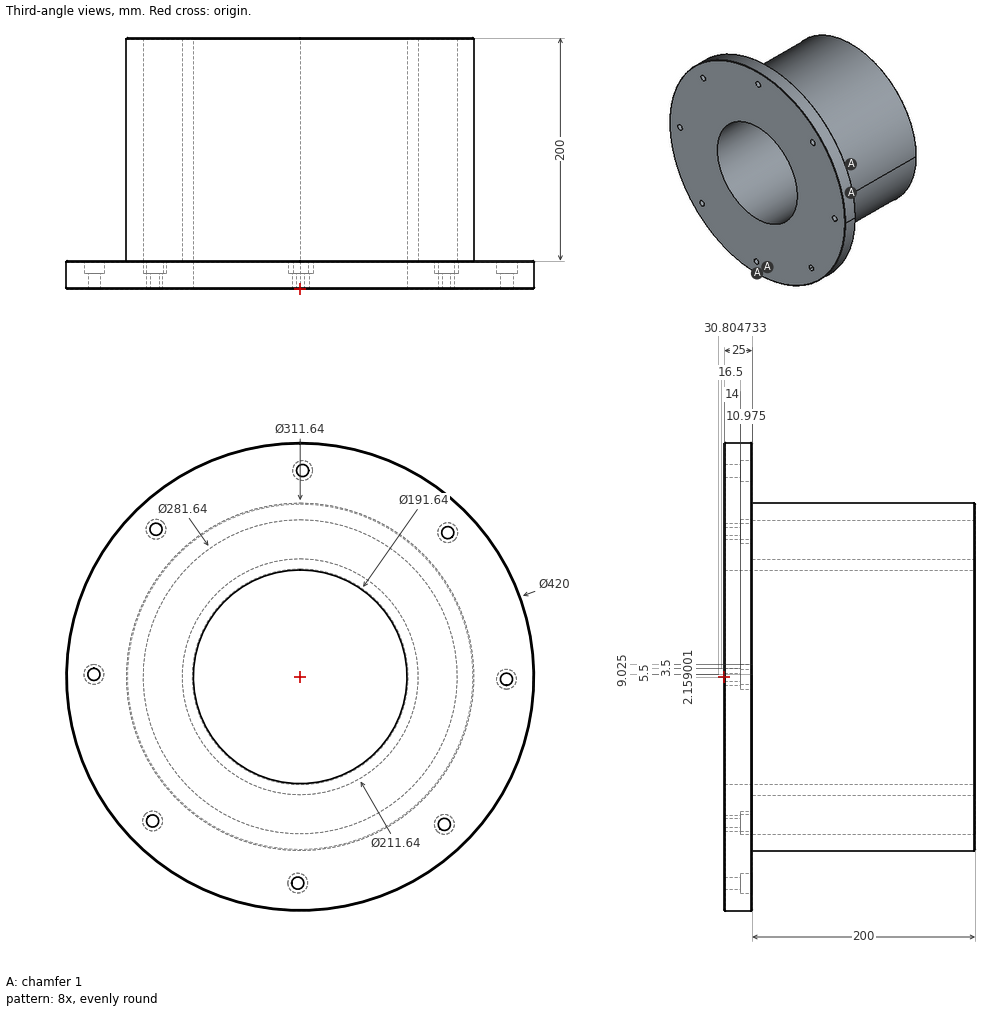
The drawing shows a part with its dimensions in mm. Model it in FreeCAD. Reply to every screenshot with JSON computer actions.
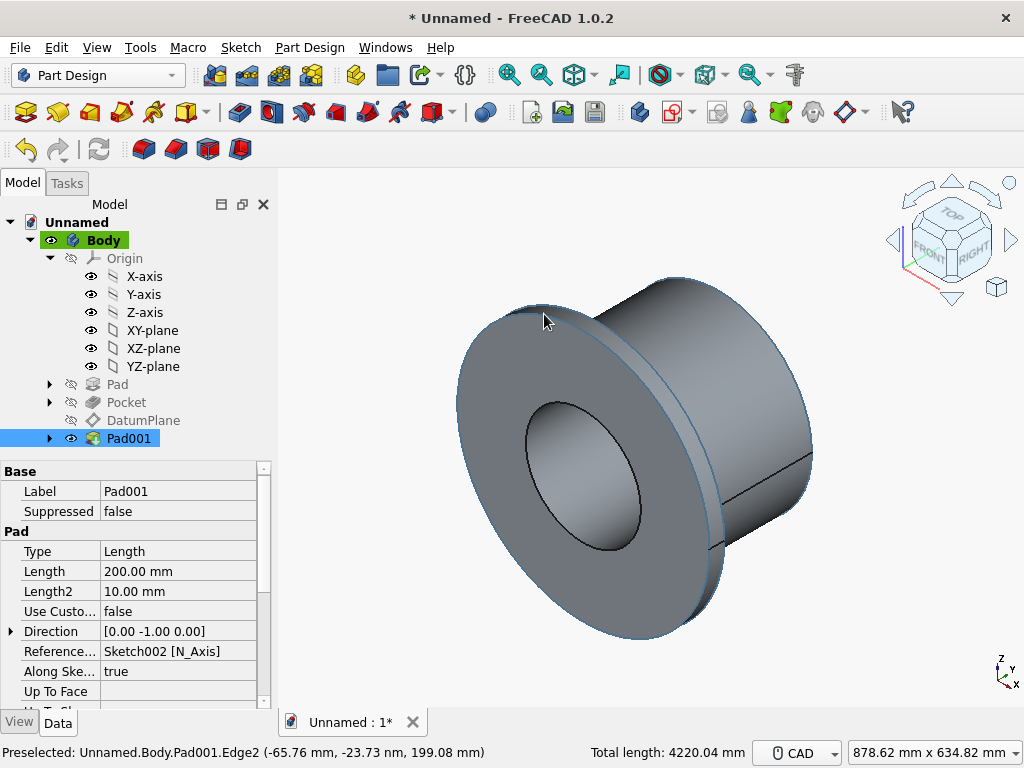
{"action": "left_click", "coordinate": [176, 150]}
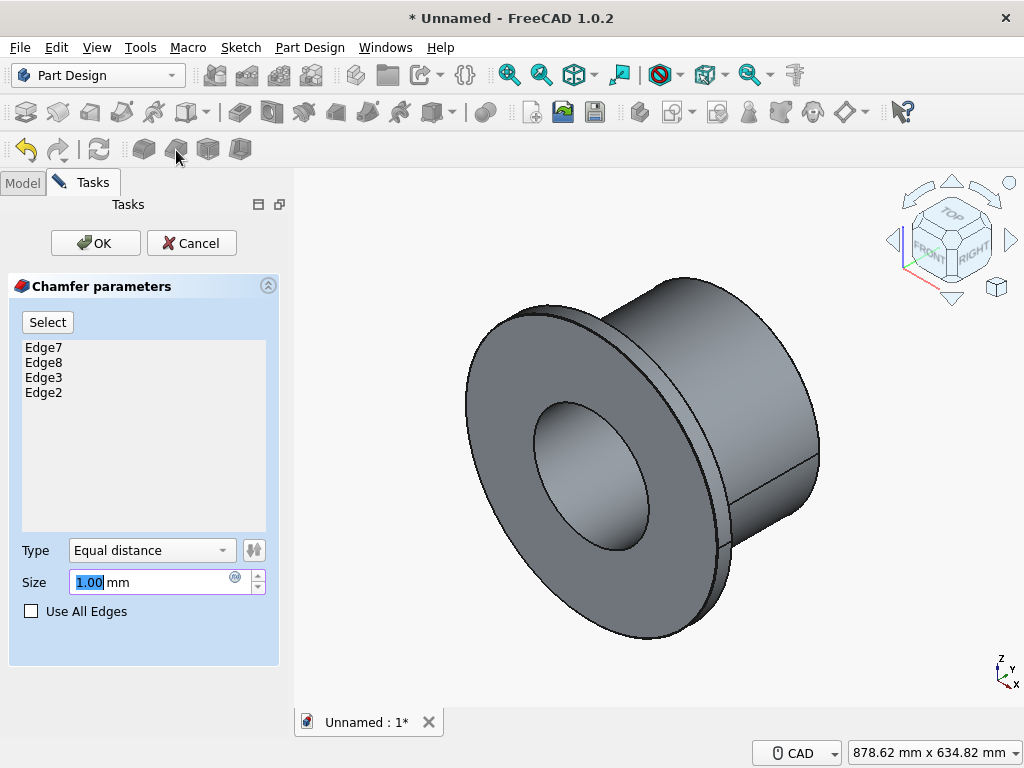
{"action": "type", "text": "1"}
{"action": "key", "text": "Tab"}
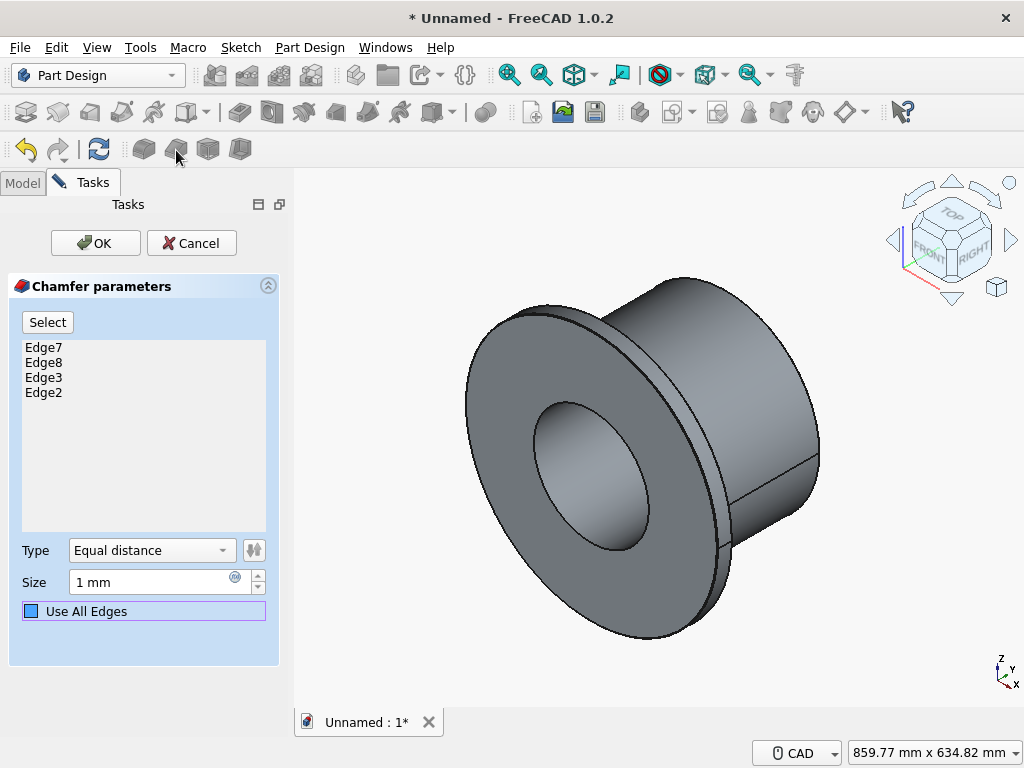
{"action": "left_click", "coordinate": [96, 243]}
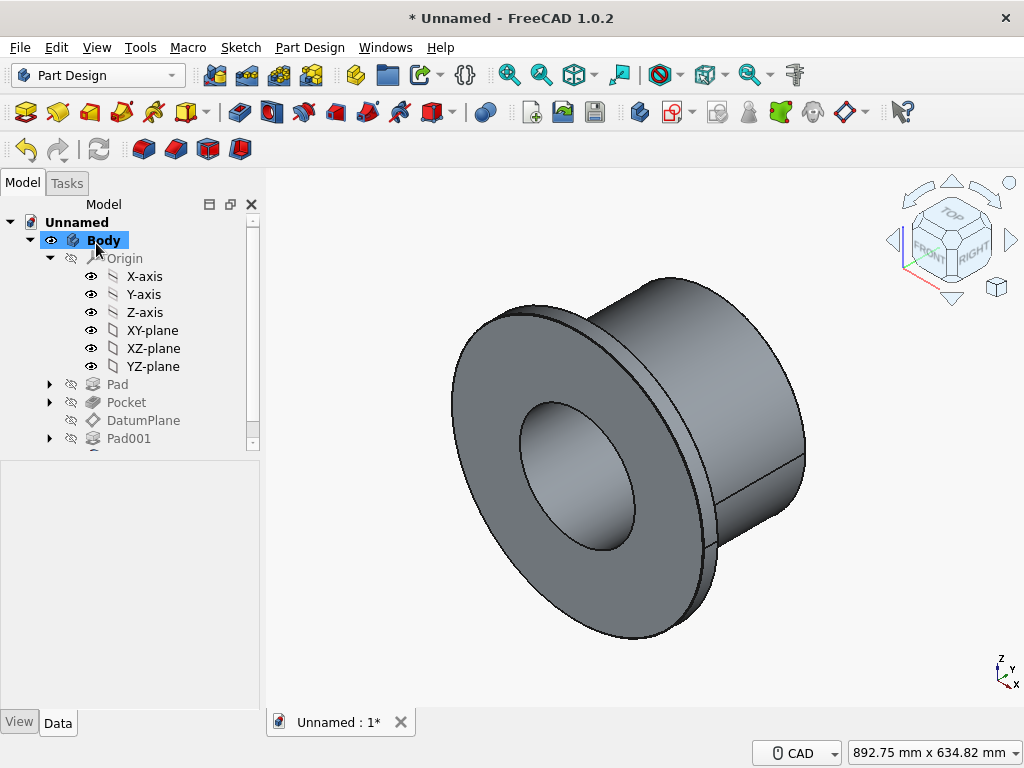
{"action": "key", "text": "4"}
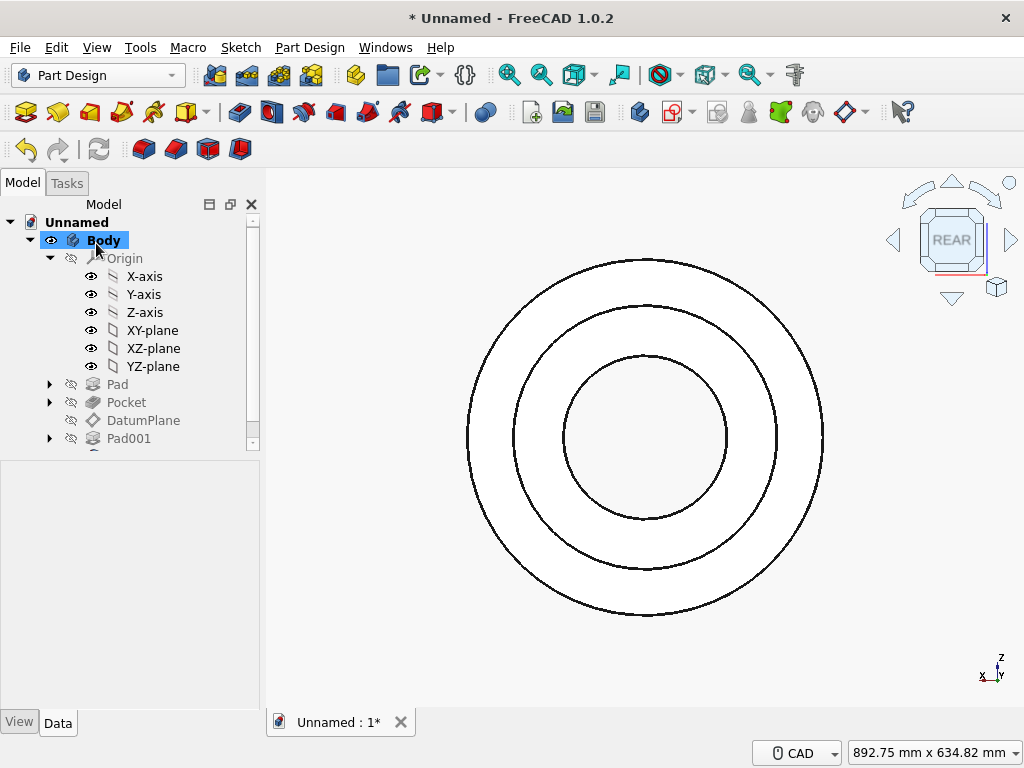
{"action": "left_click", "coordinate": [720, 361]}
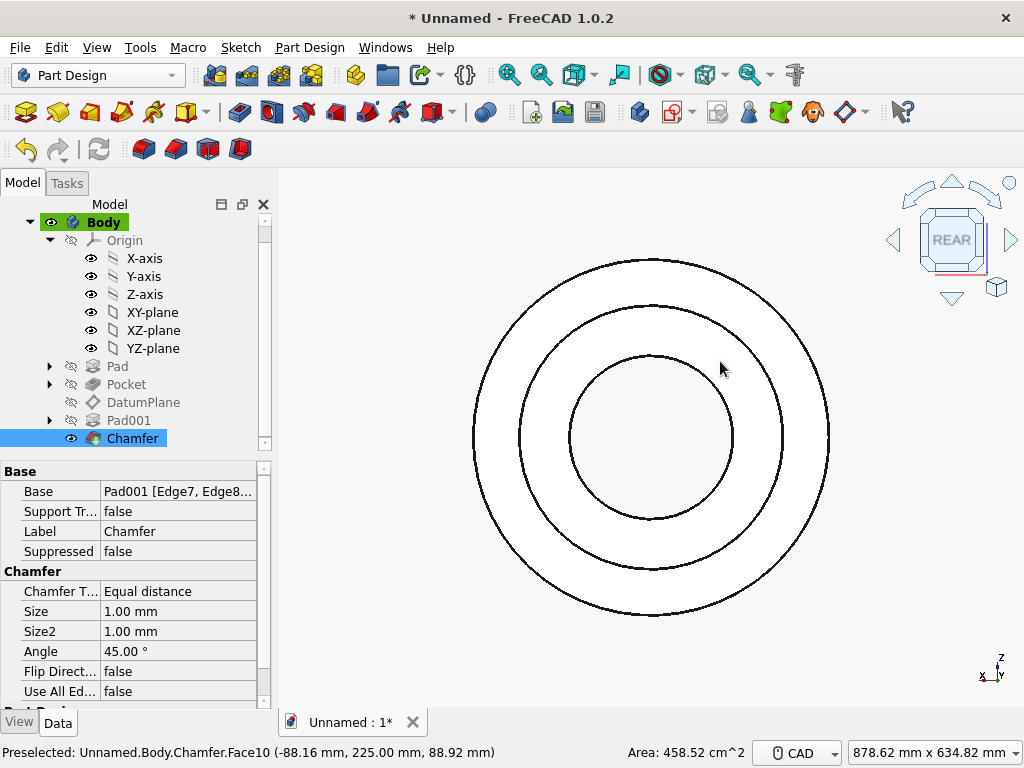
{"action": "left_click", "coordinate": [672, 112]}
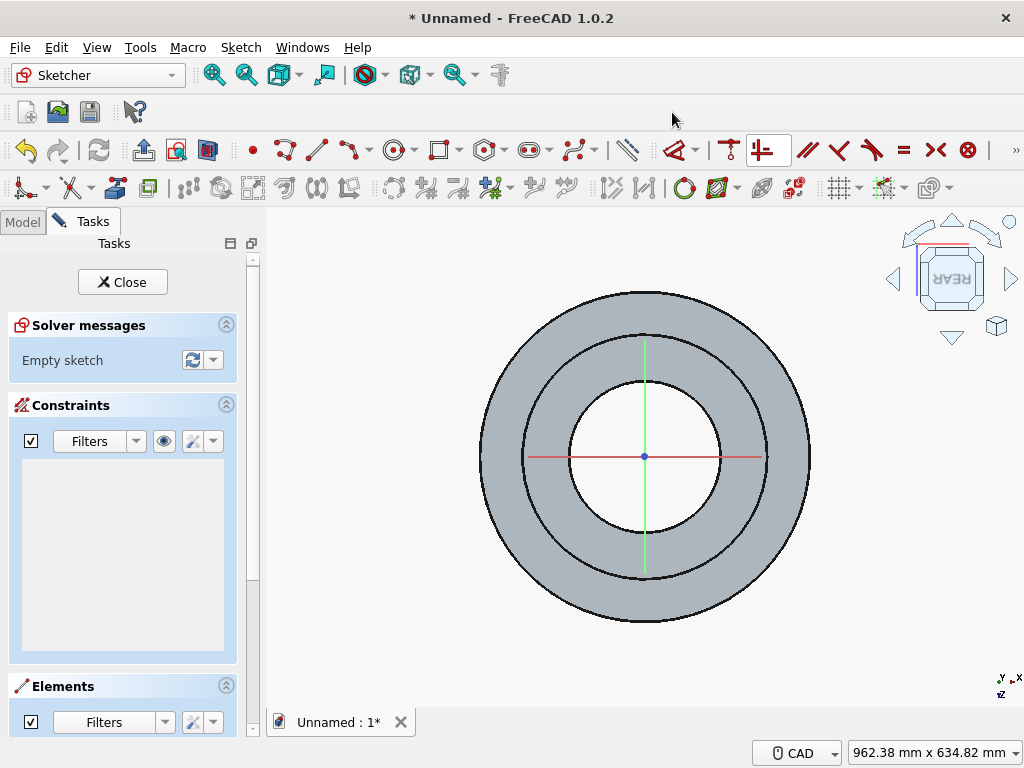
{"action": "scroll", "coordinate": [784, 457], "scroll_direction": "up", "scroll_amount": 2}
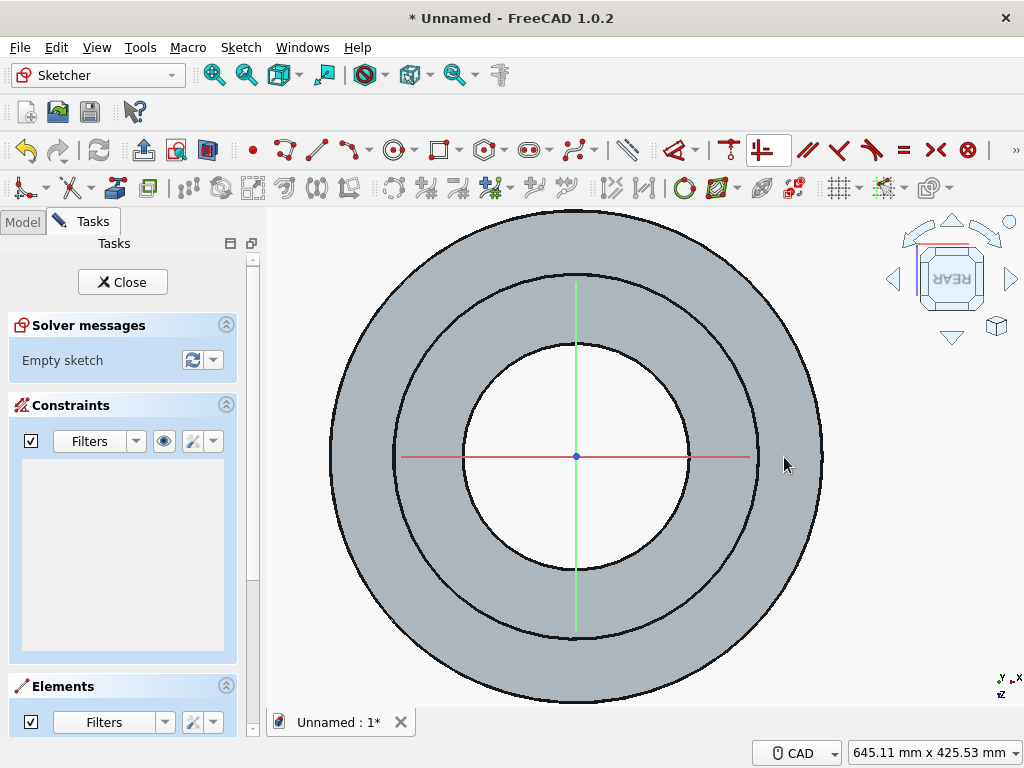
{"action": "left_click", "coordinate": [394, 150]}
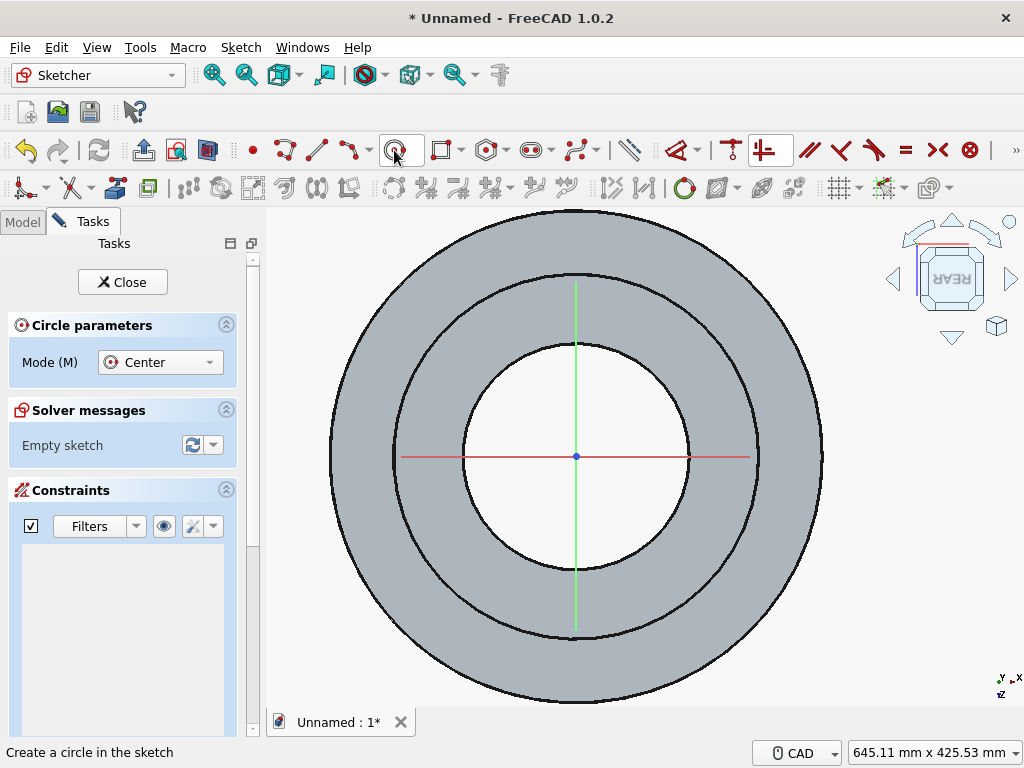
{"action": "left_click", "coordinate": [576, 457]}
{"action": "left_click", "coordinate": [693, 340]}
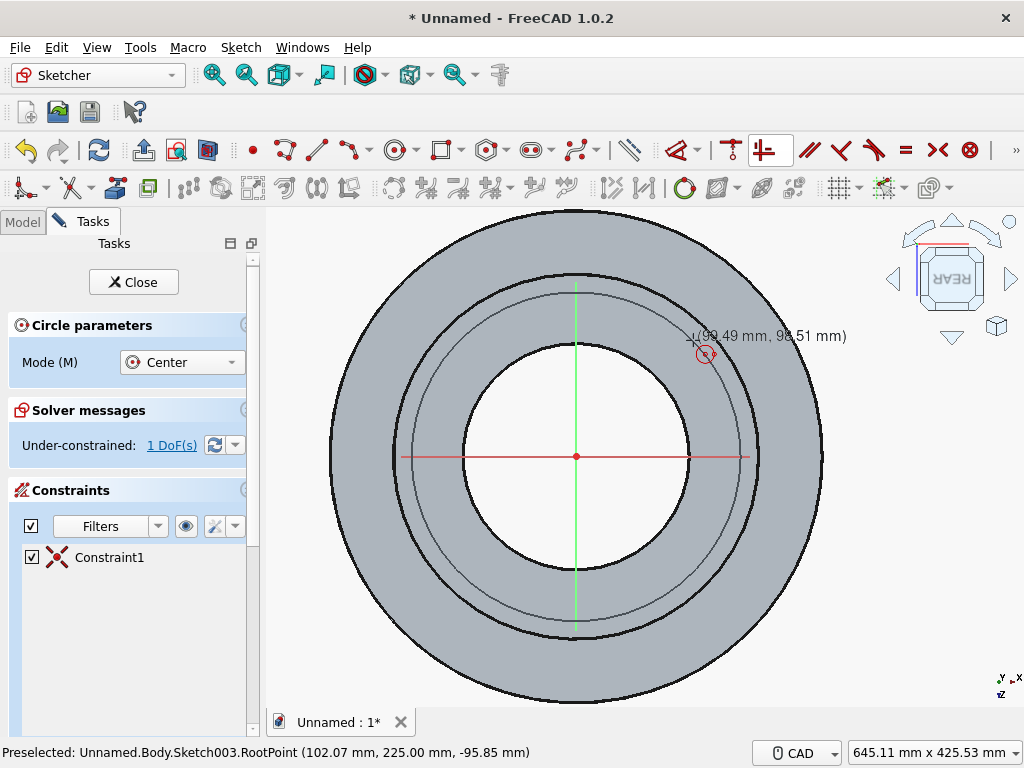
{"action": "left_click", "coordinate": [576, 457]}
{"action": "left_click", "coordinate": [664, 369]}
{"action": "key", "text": "Escape"}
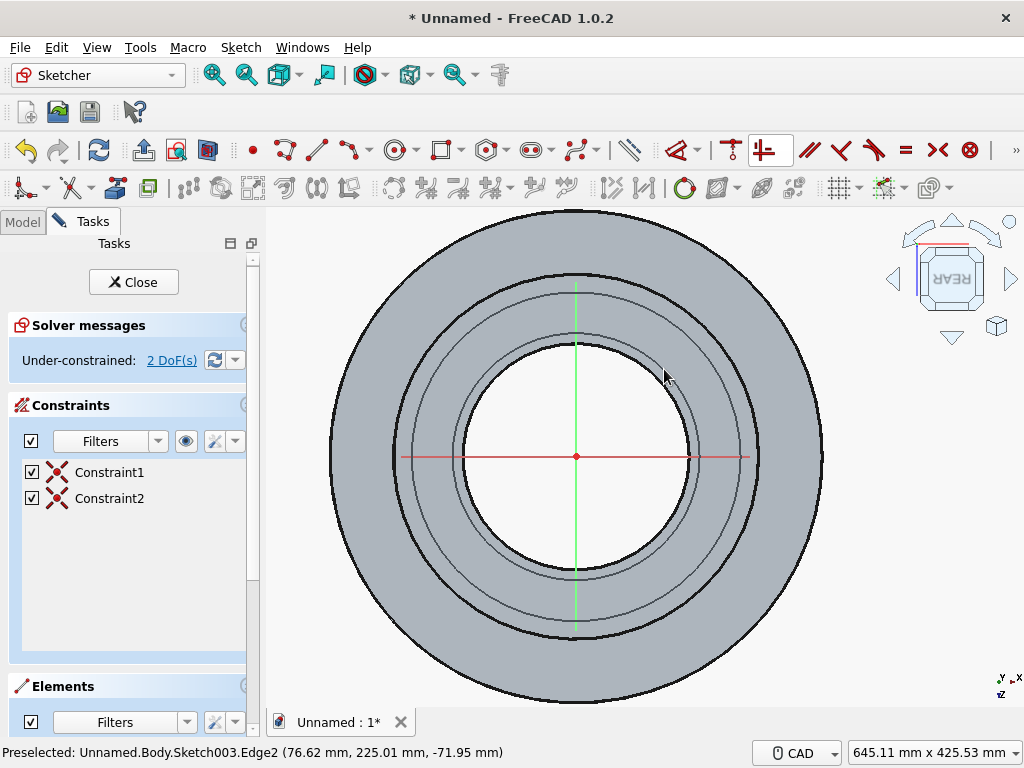
{"action": "left_click", "coordinate": [676, 150]}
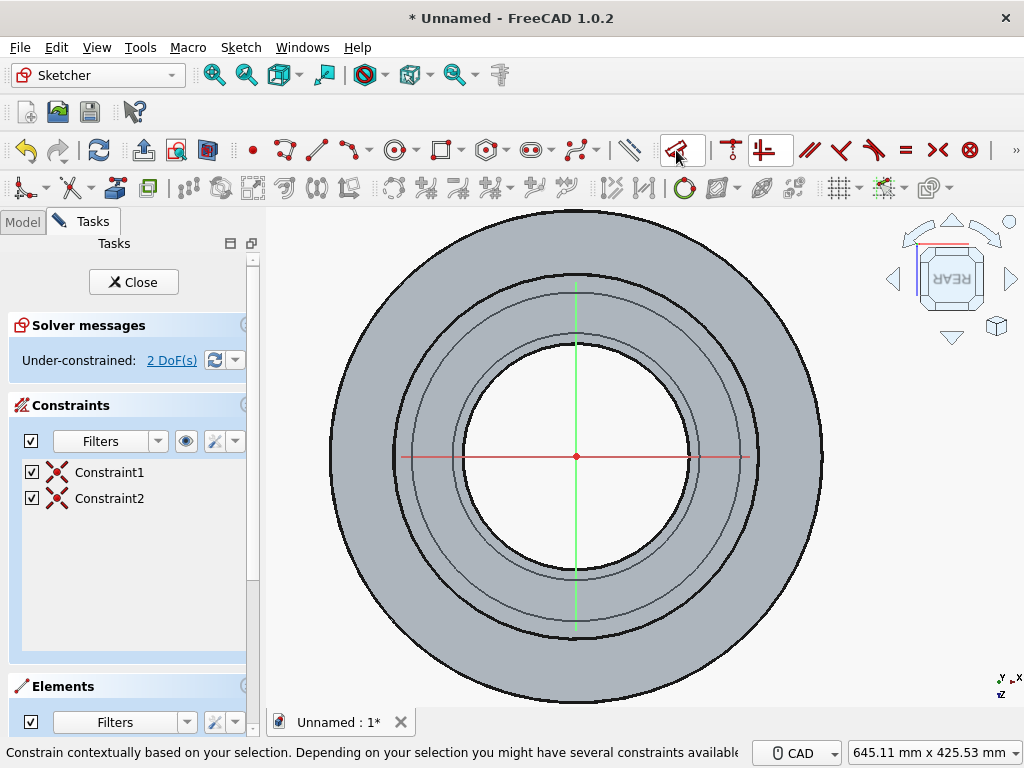
{"action": "left_click", "coordinate": [692, 340]}
{"action": "left_click", "coordinate": [715, 317]}